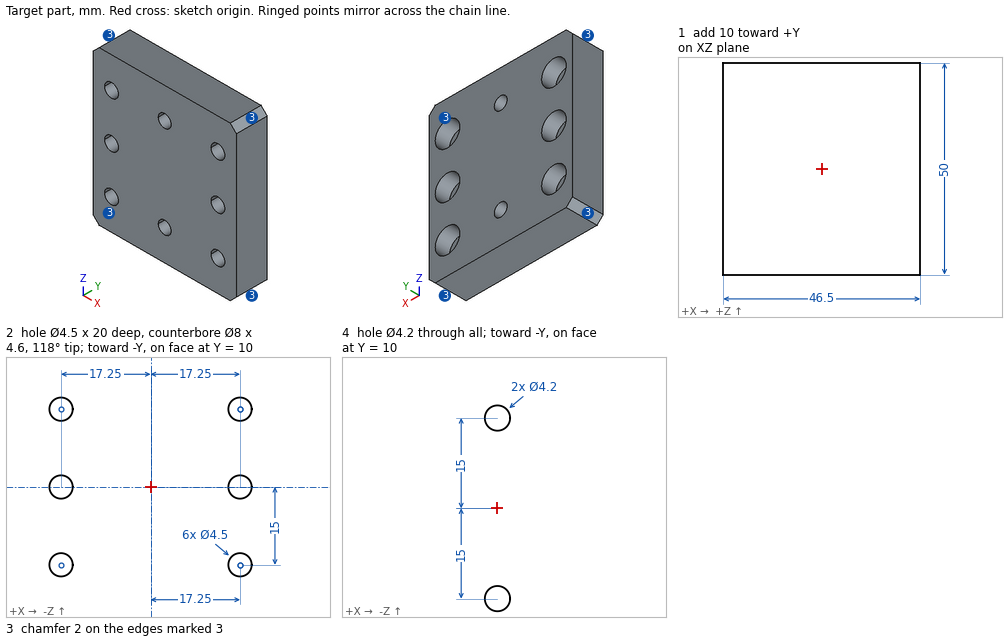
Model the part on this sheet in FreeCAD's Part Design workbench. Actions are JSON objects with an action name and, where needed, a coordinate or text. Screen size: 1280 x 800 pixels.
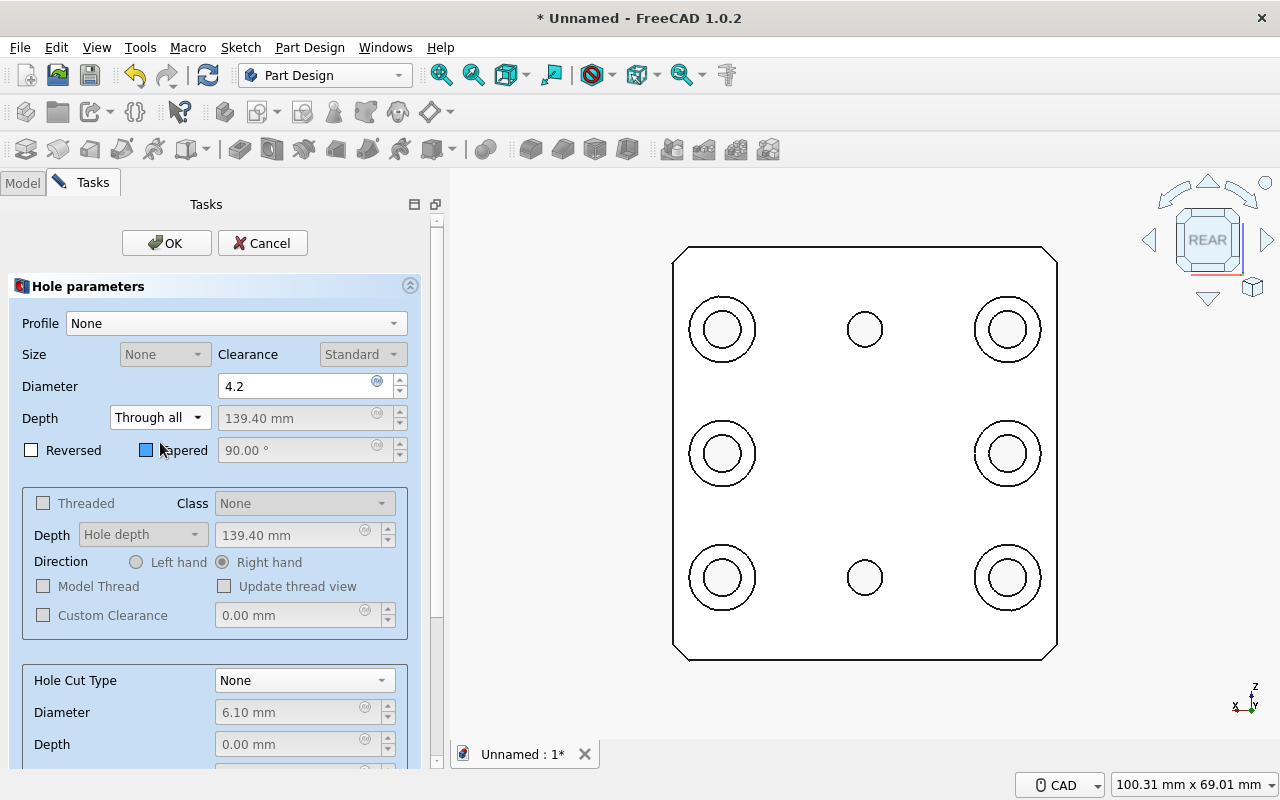
{"action": "left_click", "coordinate": [167, 243]}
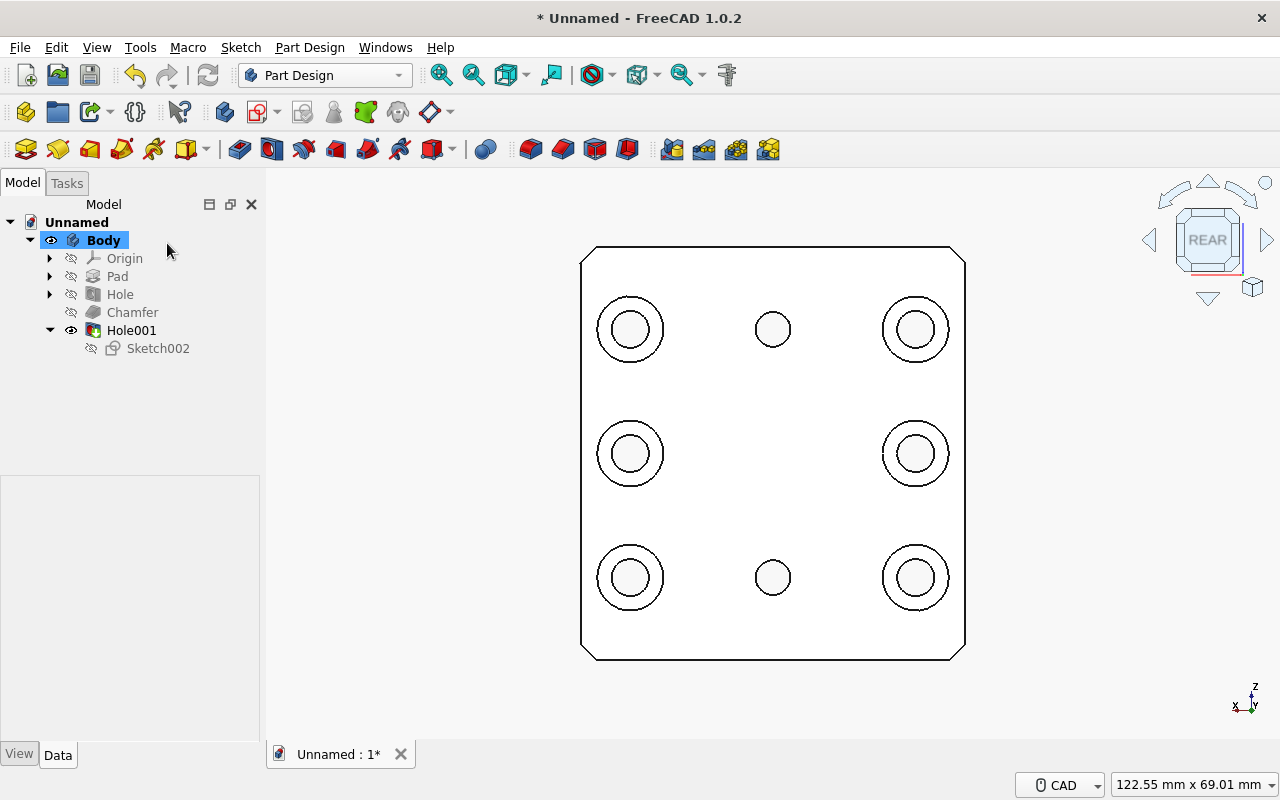
{"action": "key", "text": "0"}